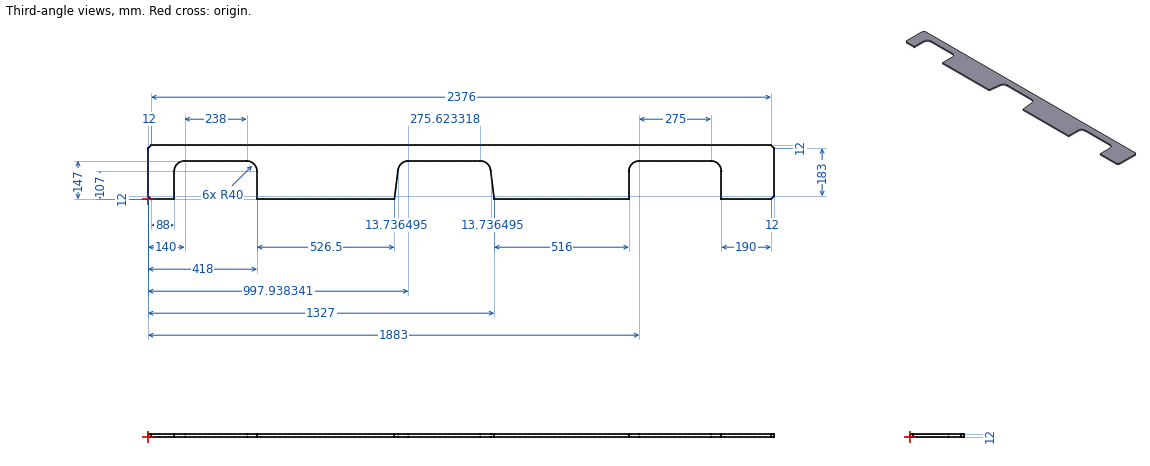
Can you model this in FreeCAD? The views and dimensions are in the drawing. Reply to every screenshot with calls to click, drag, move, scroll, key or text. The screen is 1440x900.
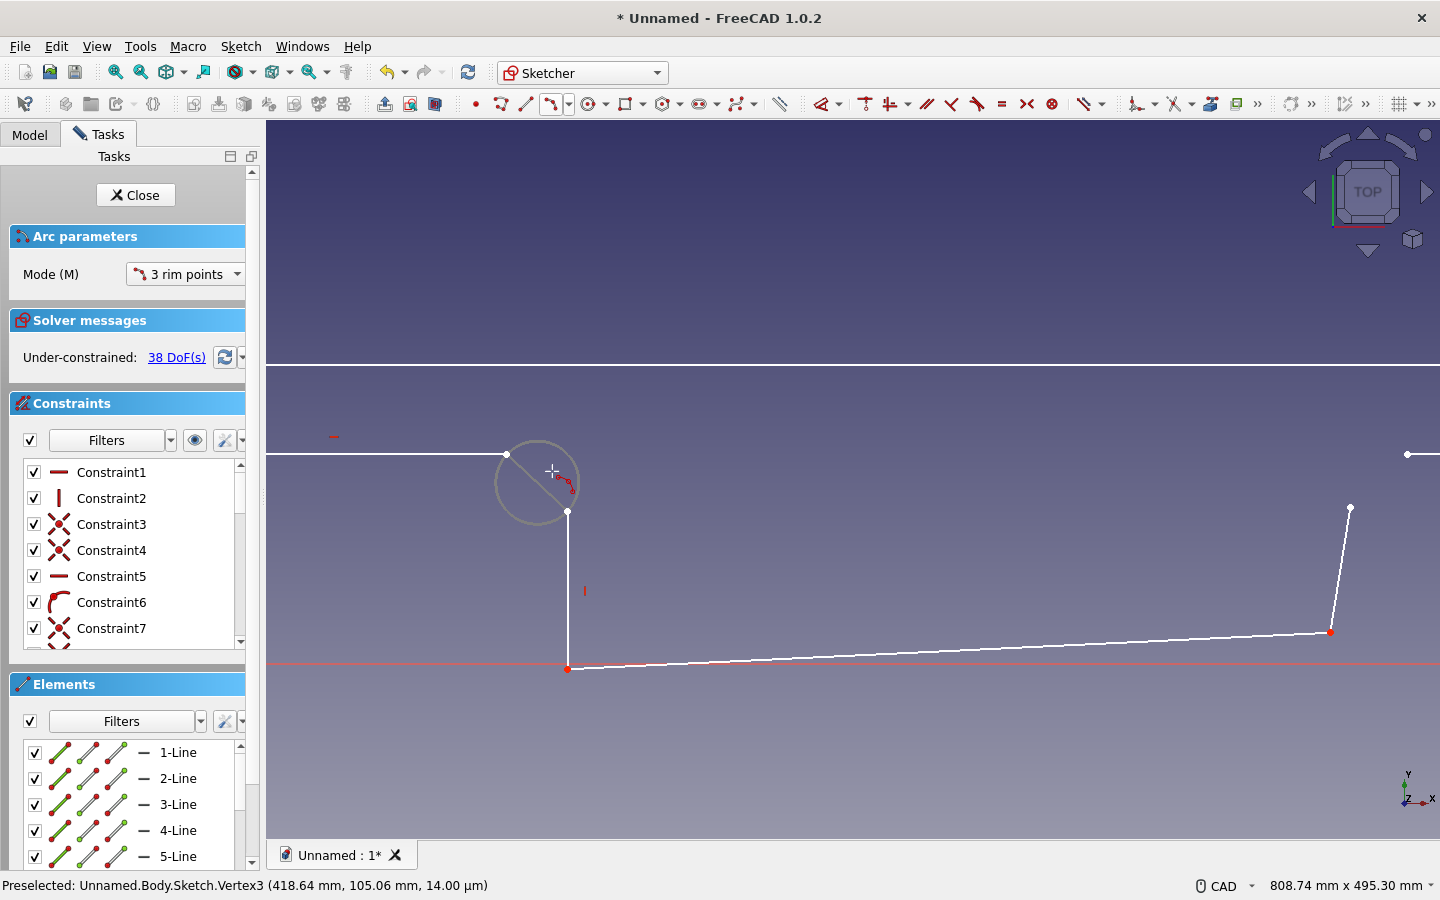
click(550, 467)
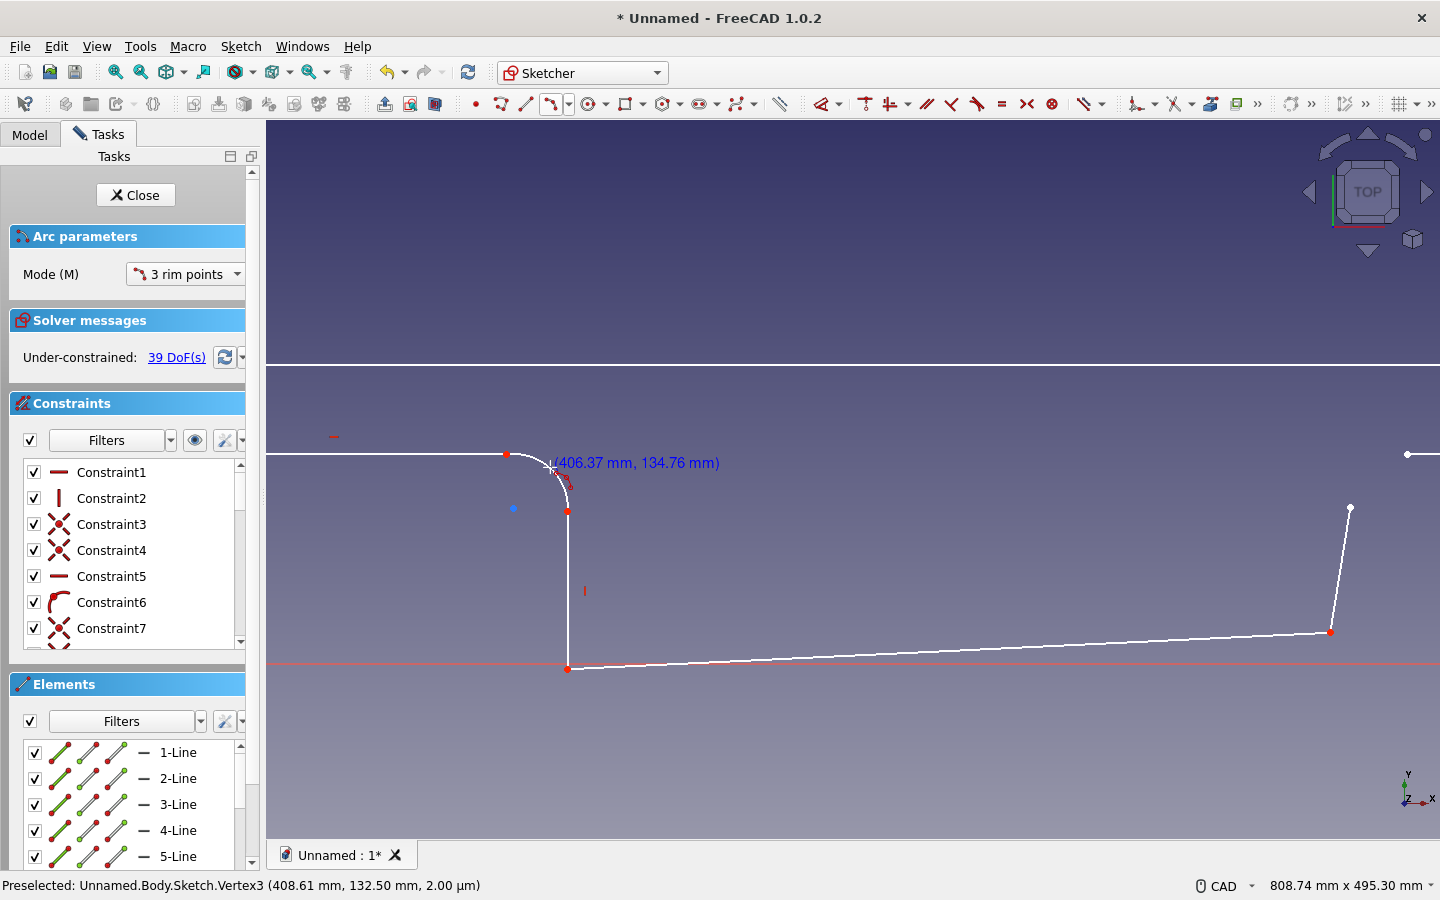
scroll(552, 471, down, 8)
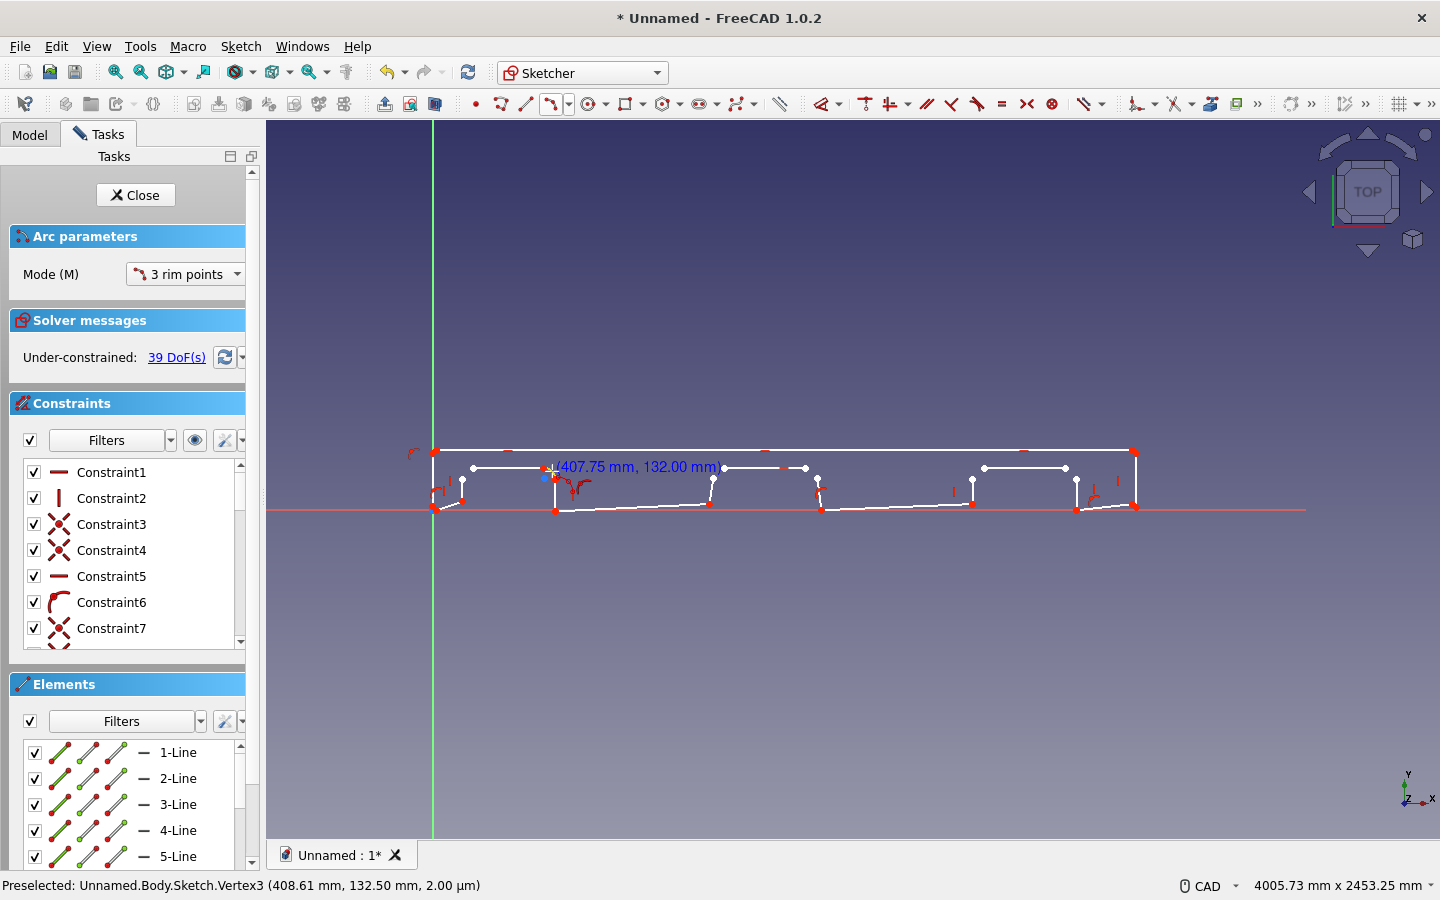
click(713, 479)
click(725, 468)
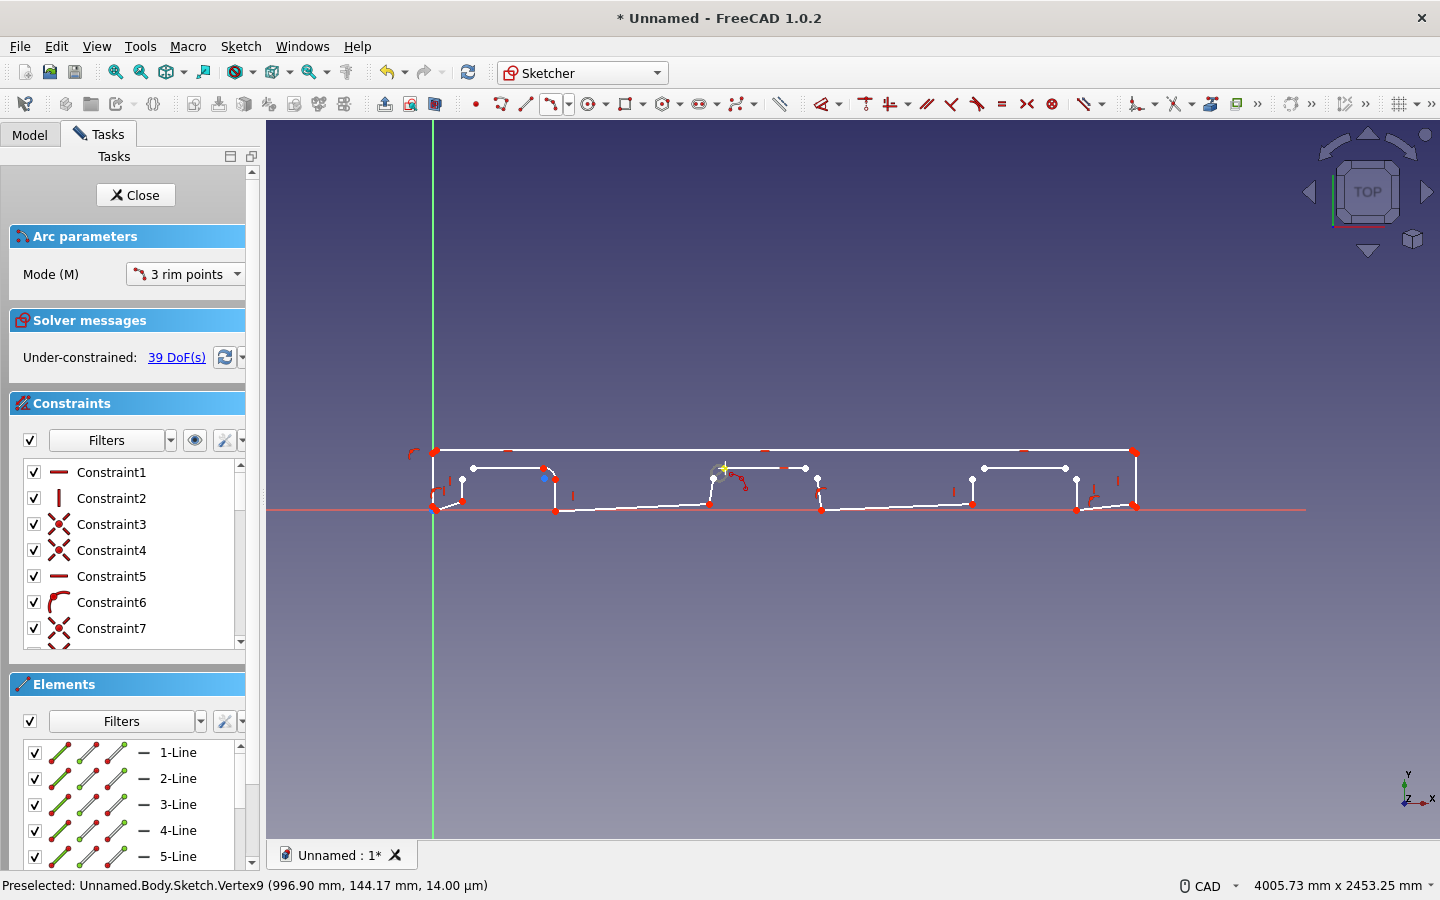
scroll(717, 470, up, 9)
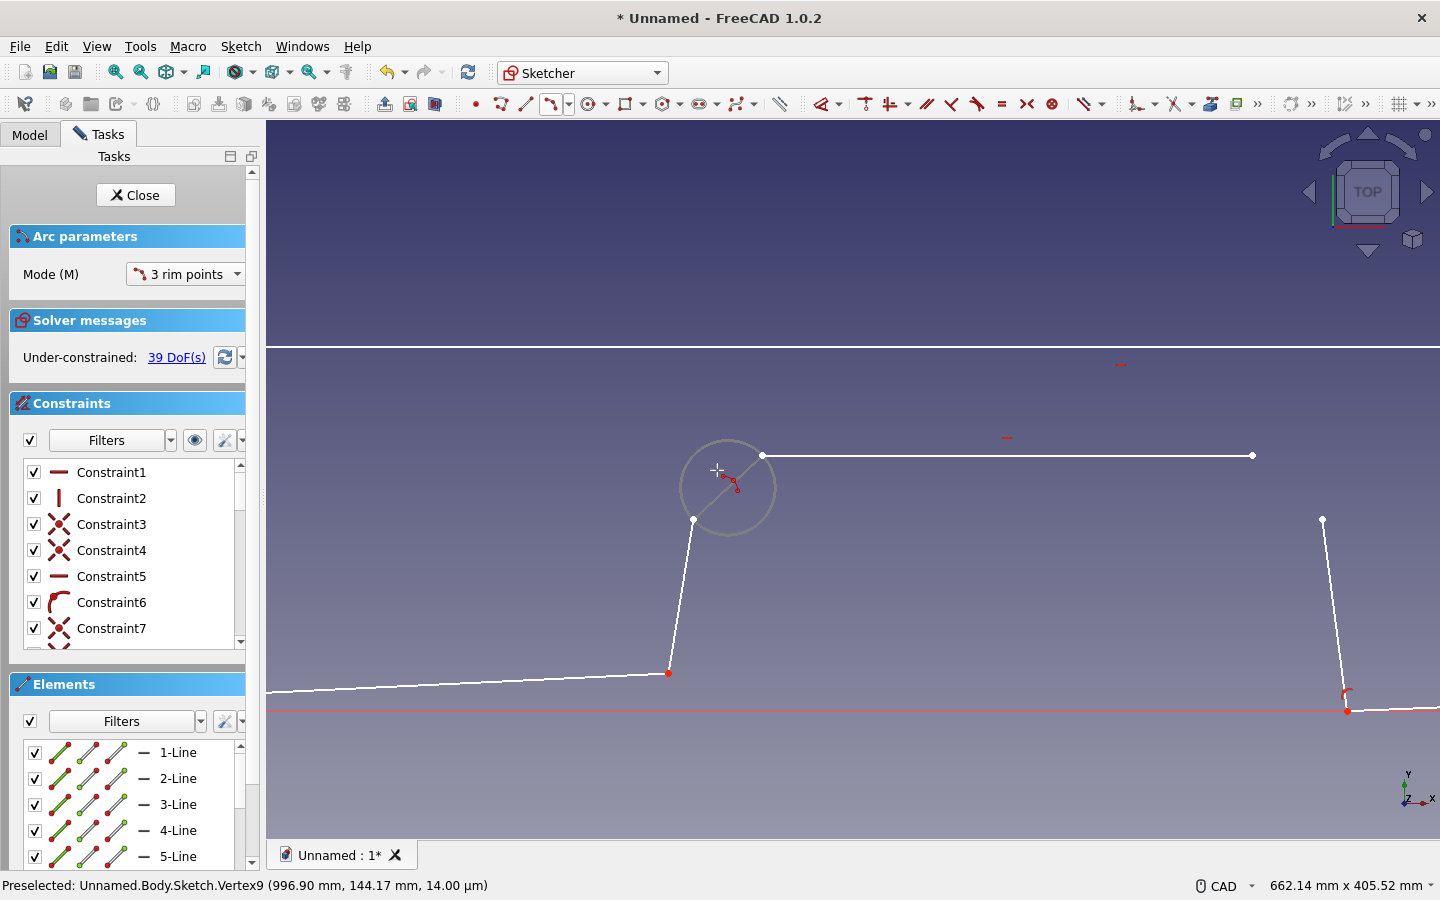
click(717, 468)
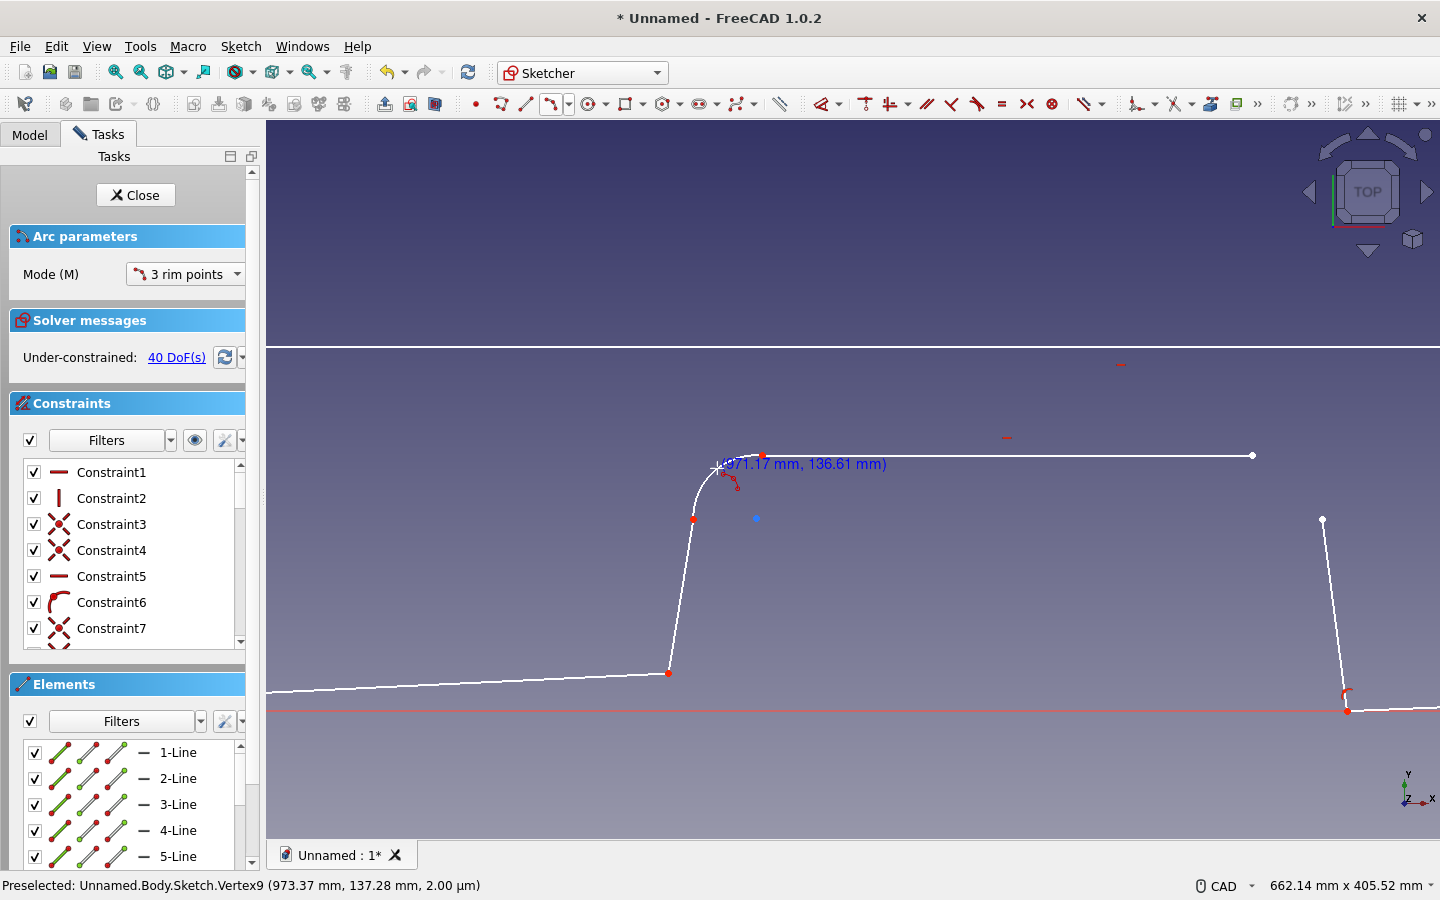
scroll(718, 470, down, 9)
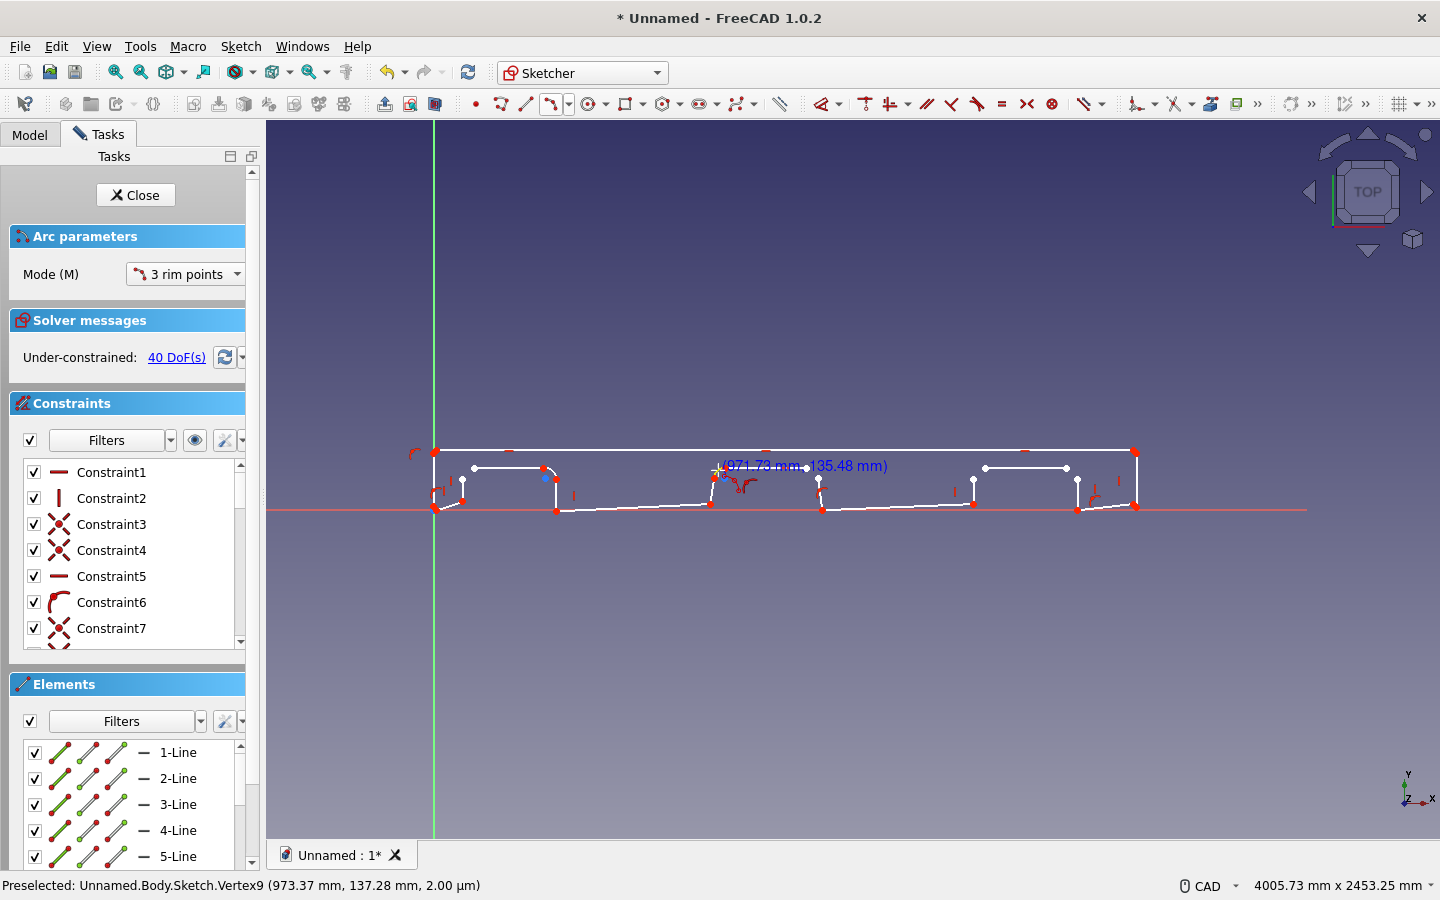
click(807, 468)
click(818, 479)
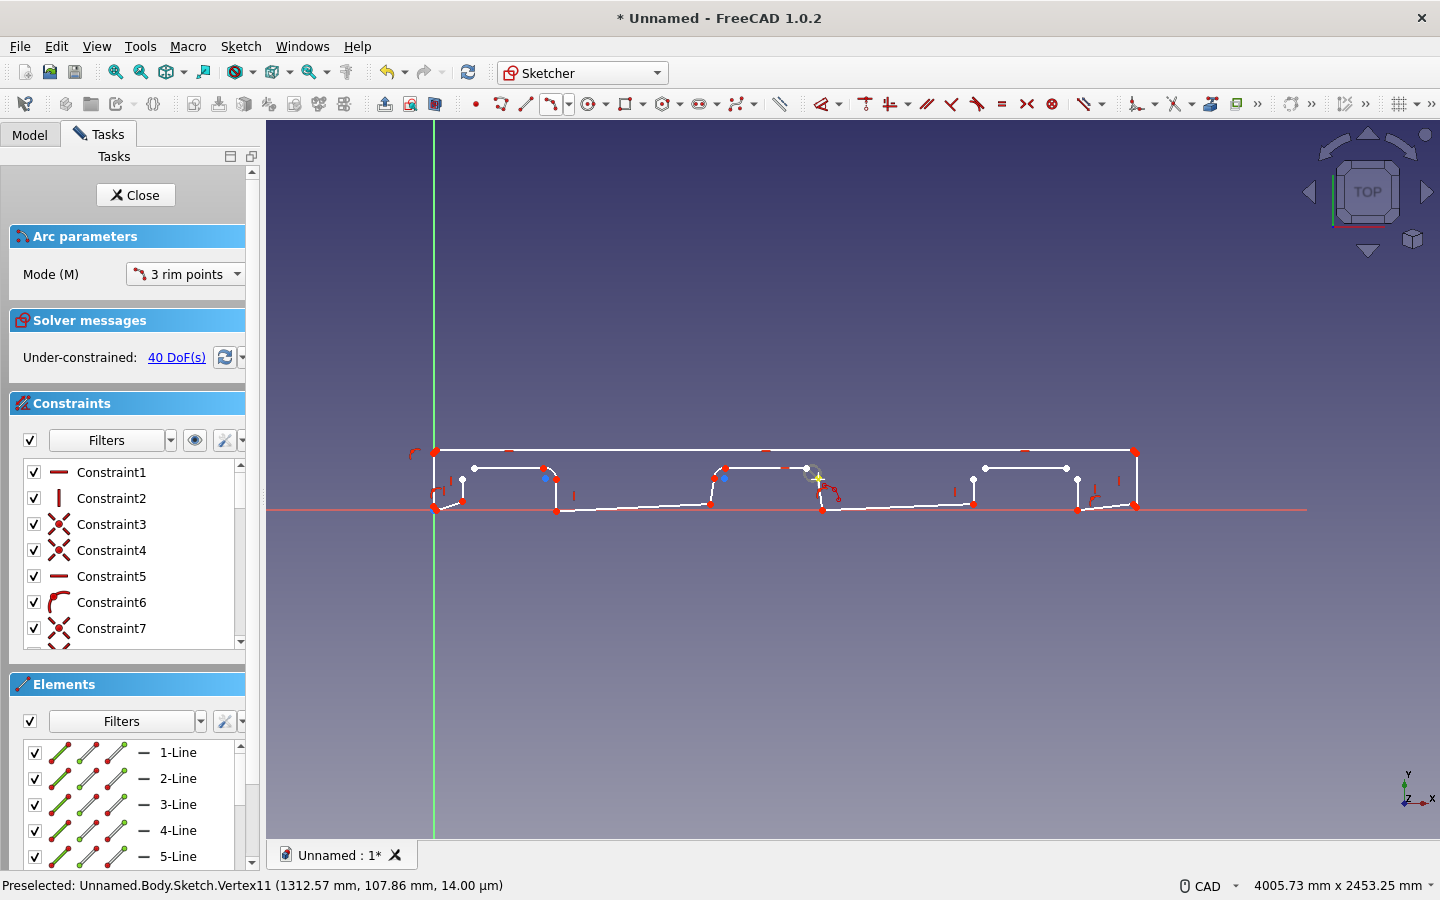
scroll(815, 470, up, 9)